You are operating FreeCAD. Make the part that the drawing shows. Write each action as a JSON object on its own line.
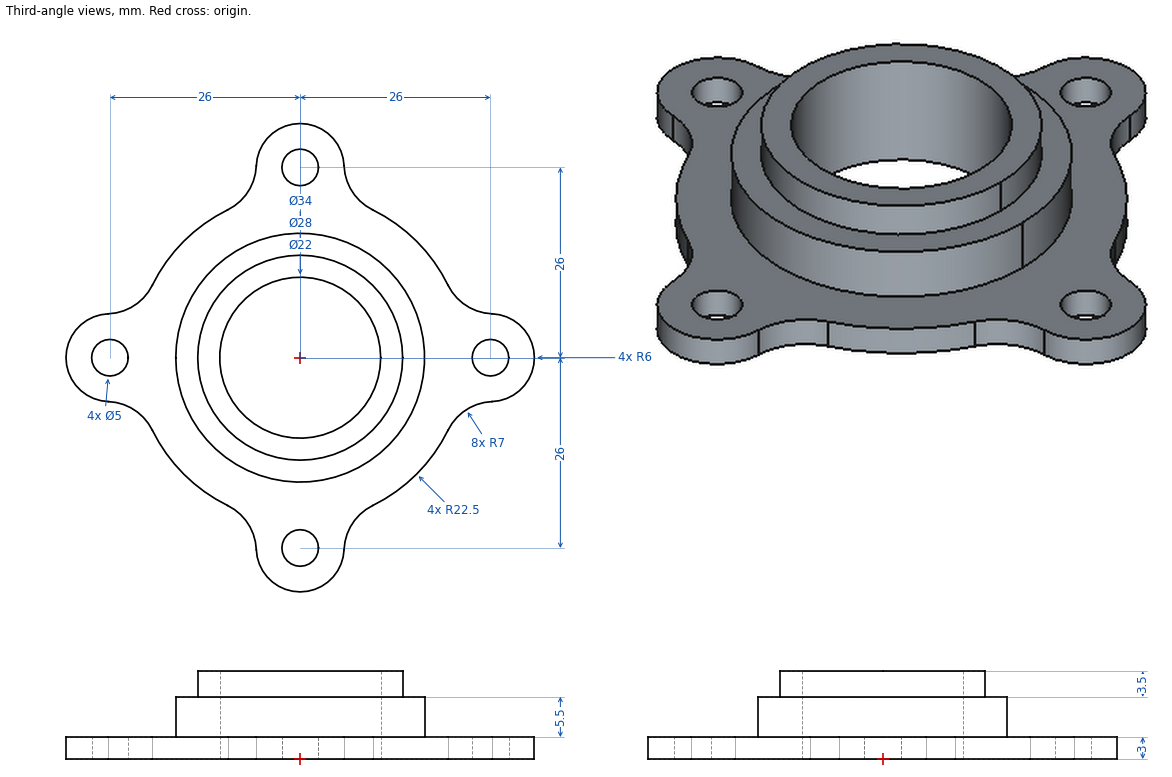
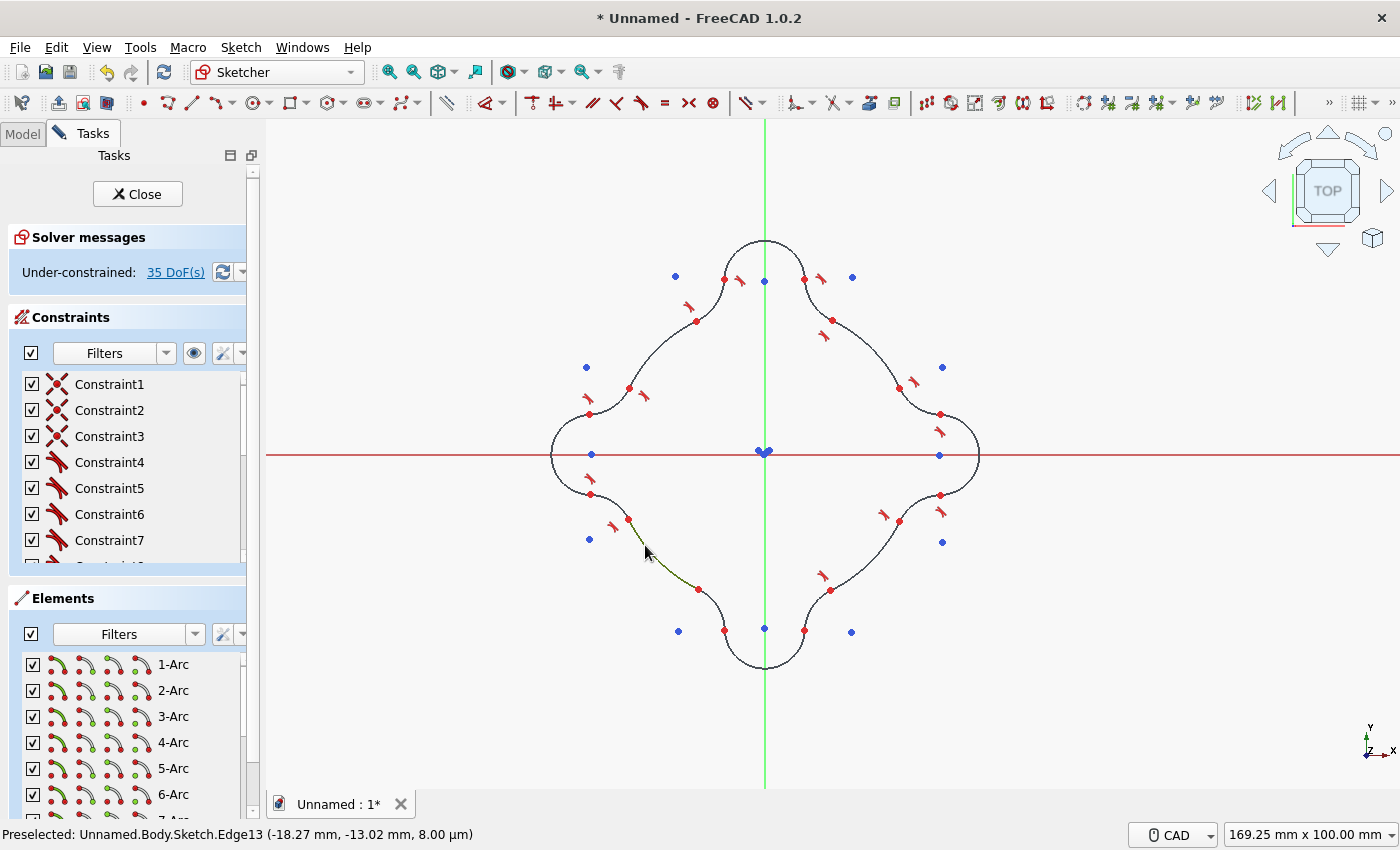
{"action": "left_click", "coordinate": [722, 616]}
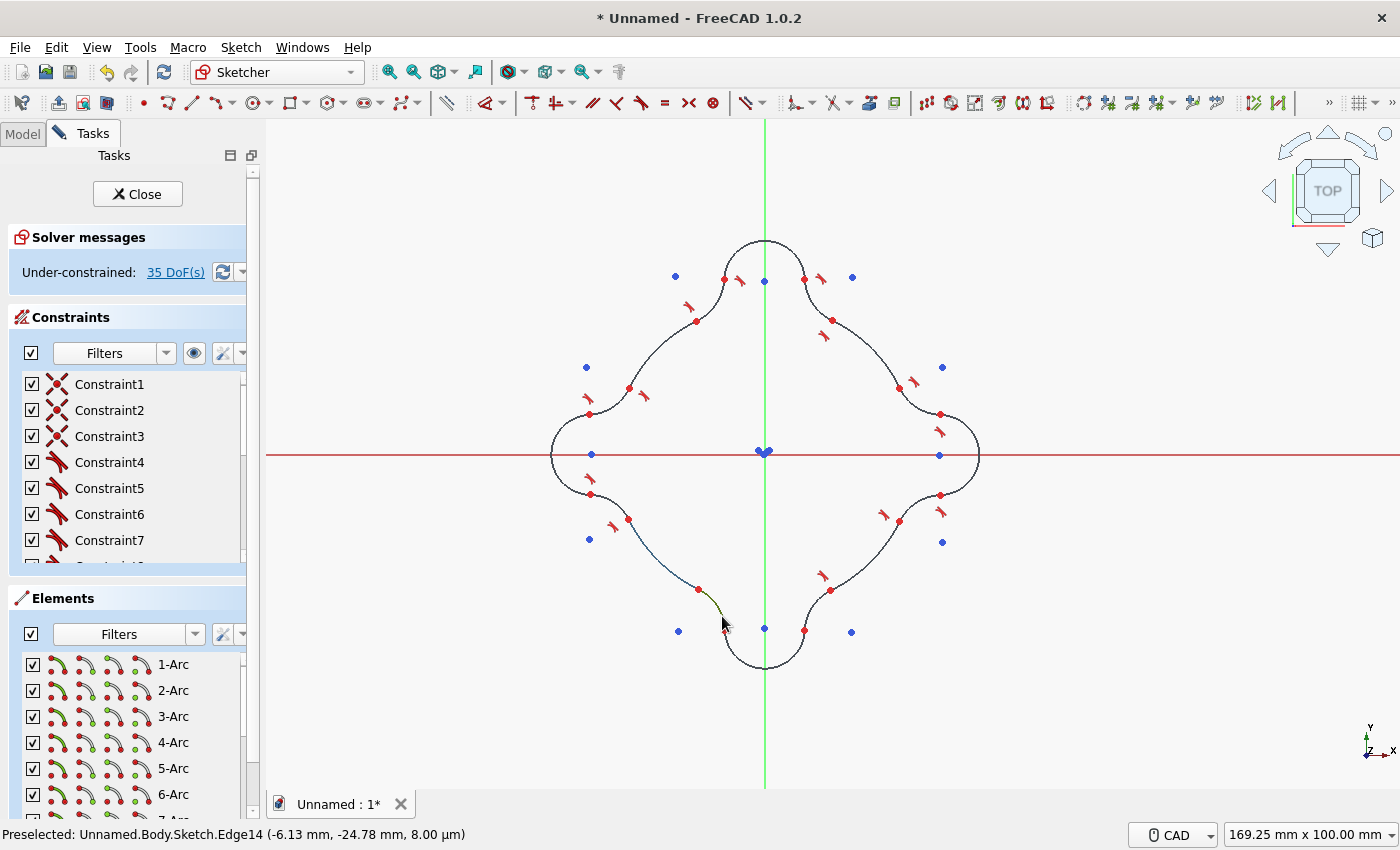
{"action": "left_click", "coordinate": [642, 104]}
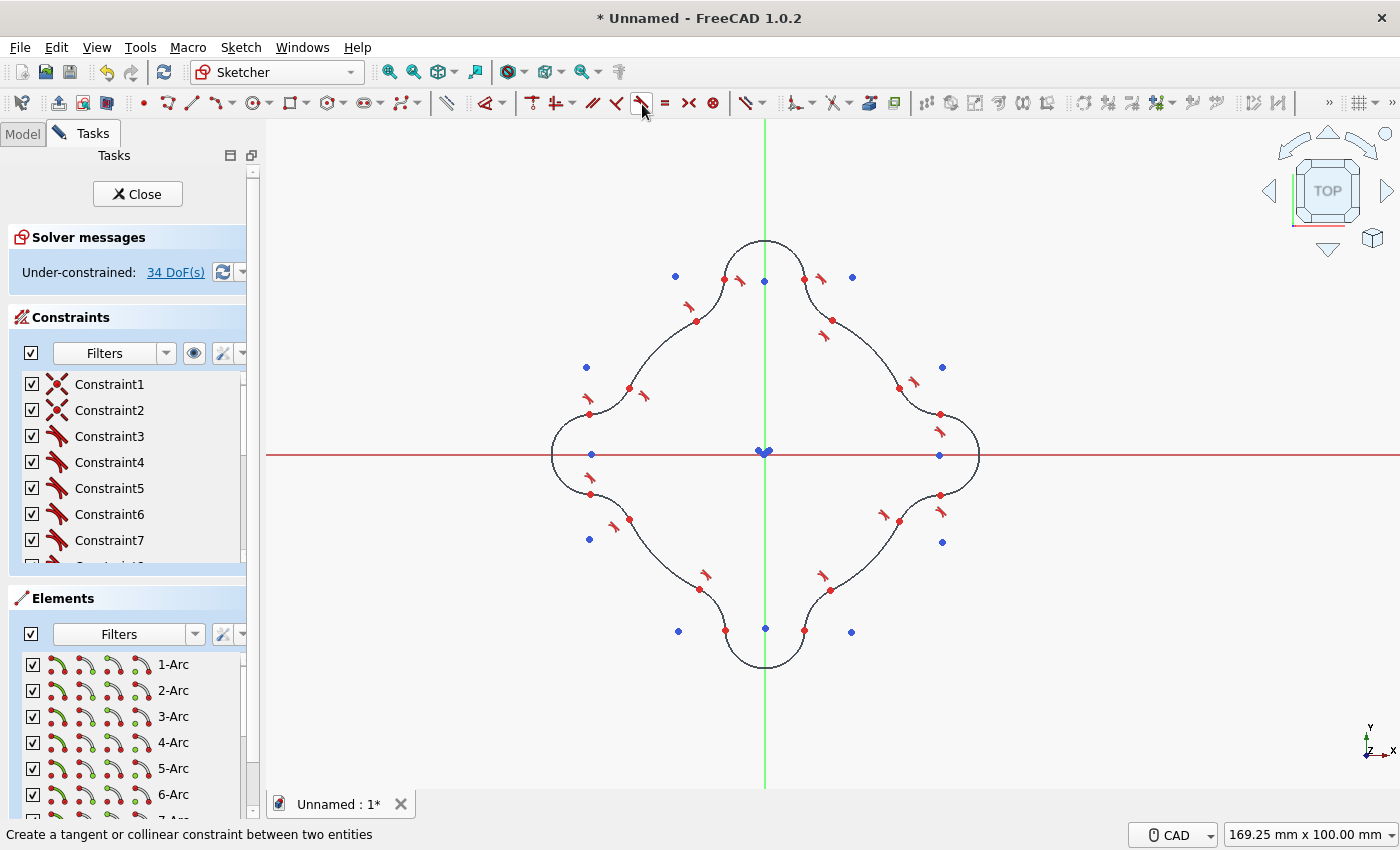
{"action": "left_click", "coordinate": [723, 616]}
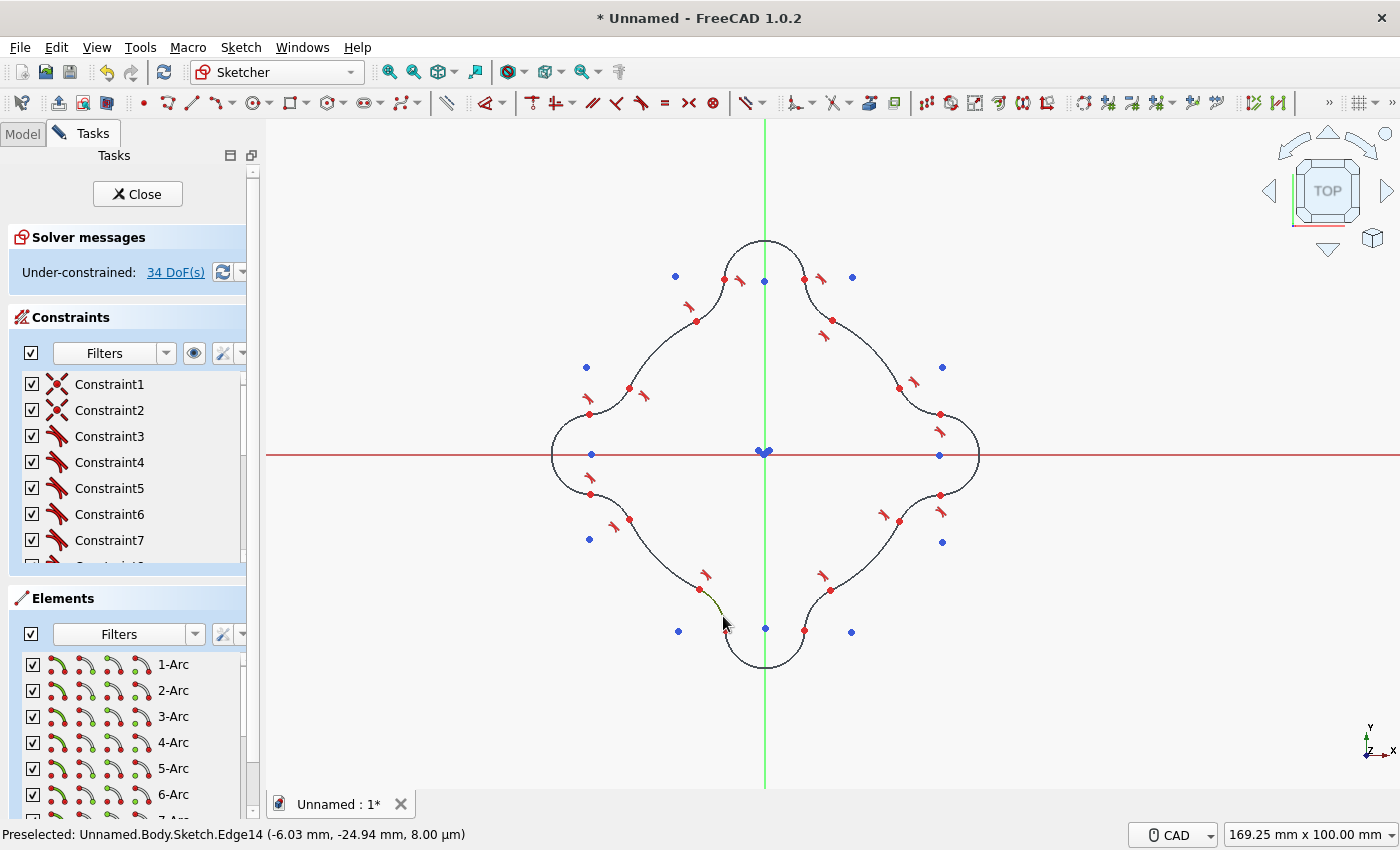
{"action": "left_click", "coordinate": [742, 661]}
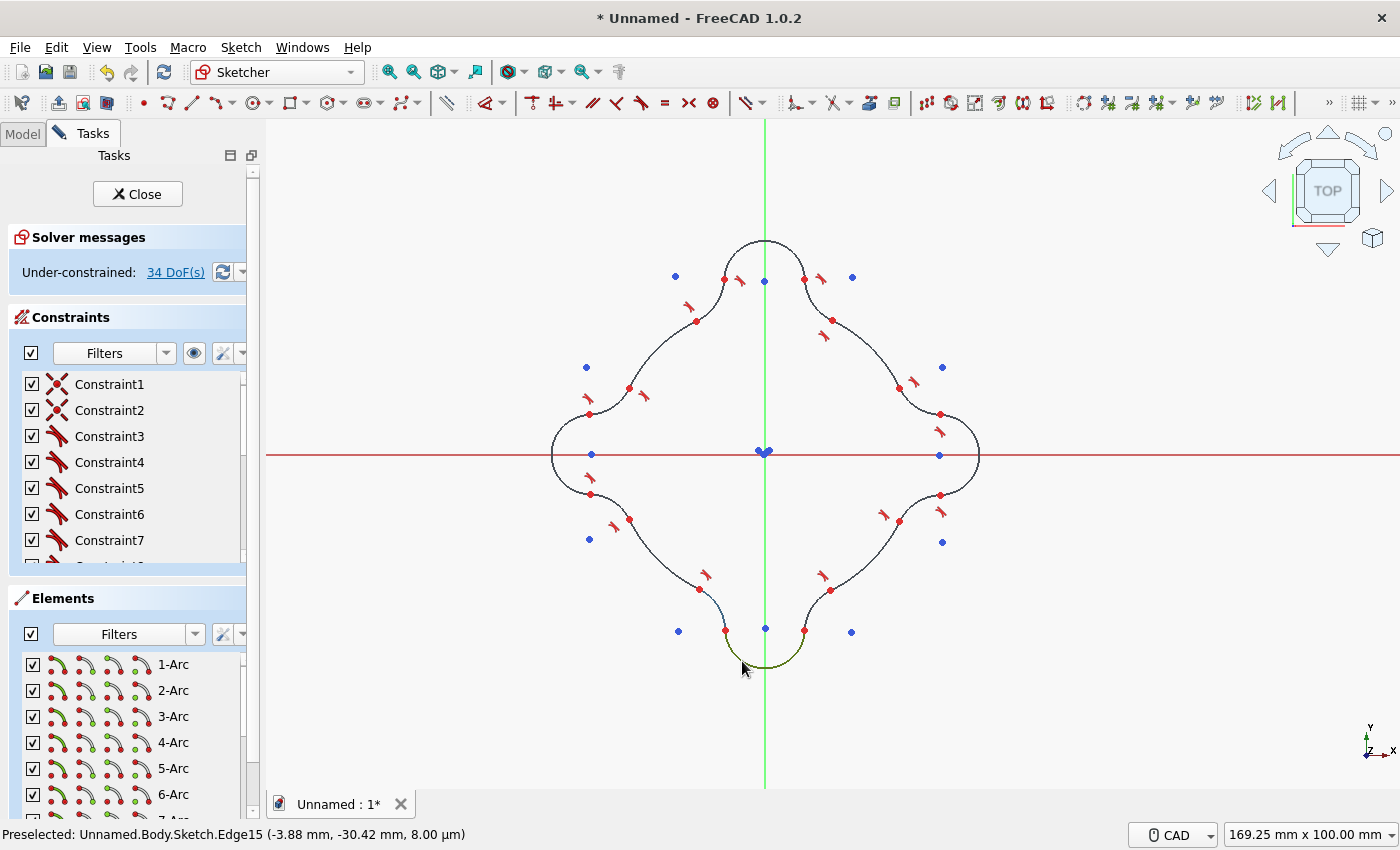
{"action": "left_click", "coordinate": [642, 104]}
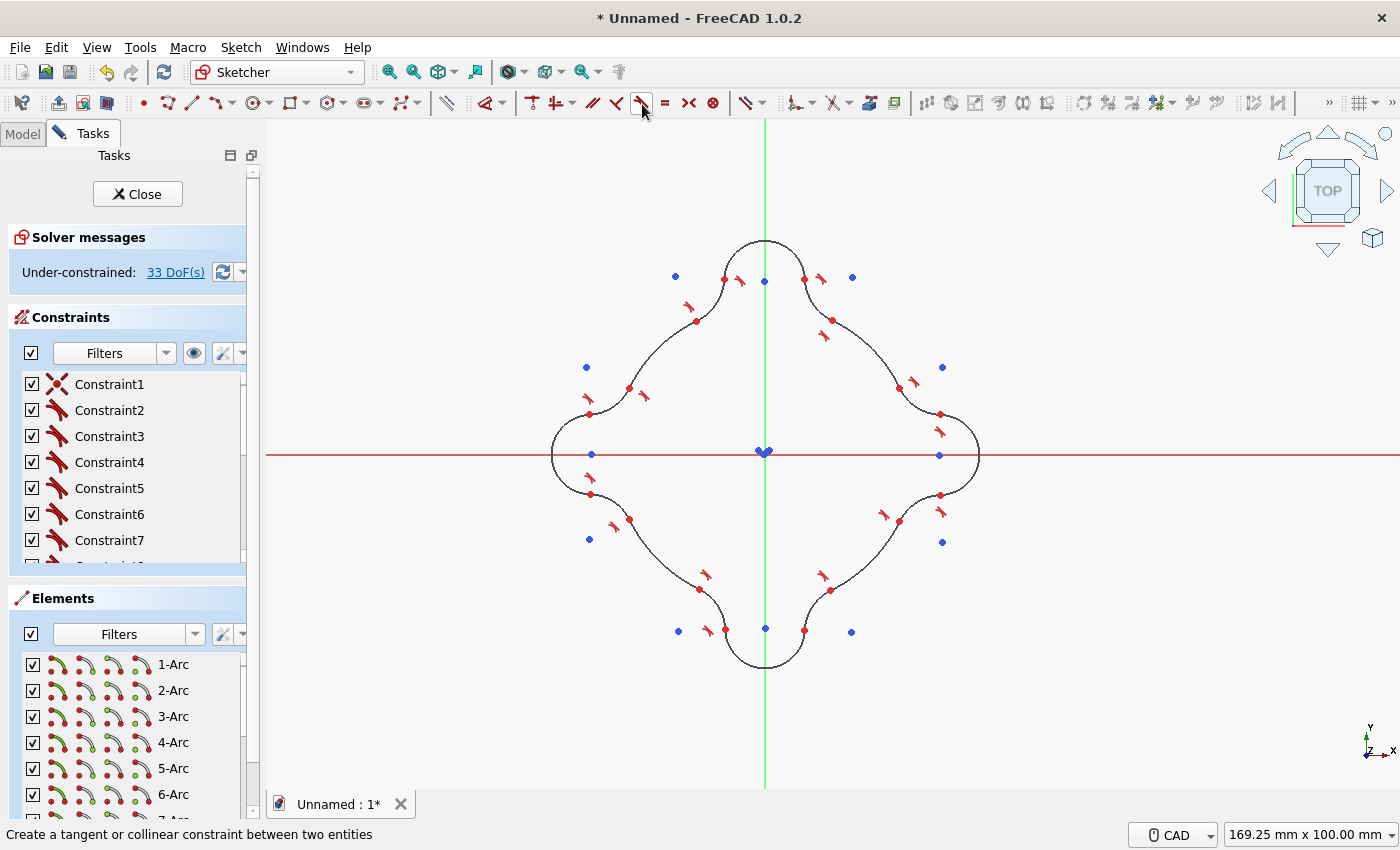
{"action": "left_click", "coordinate": [742, 661]}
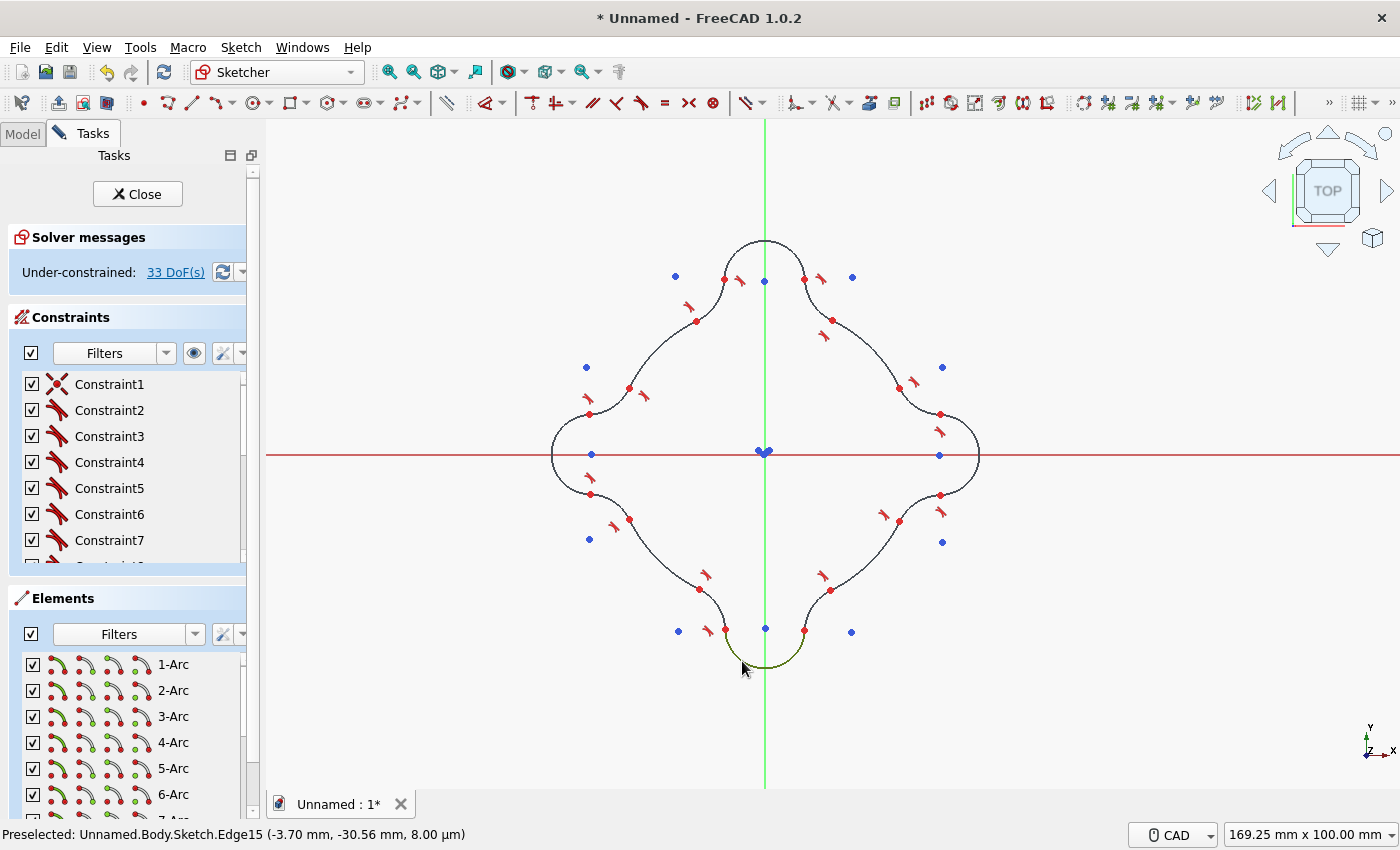
{"action": "left_click", "coordinate": [819, 599]}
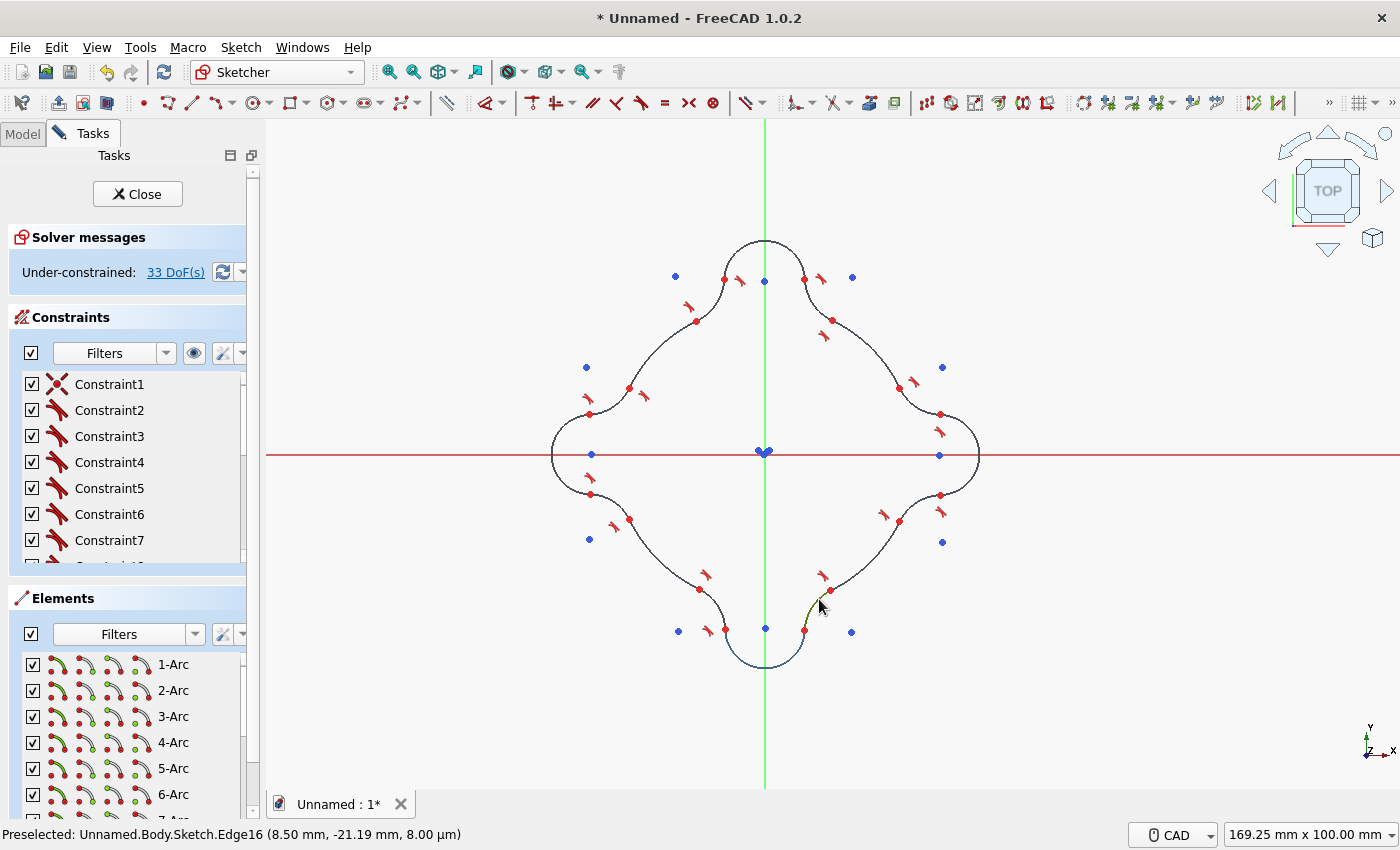
{"action": "left_click", "coordinate": [642, 104]}